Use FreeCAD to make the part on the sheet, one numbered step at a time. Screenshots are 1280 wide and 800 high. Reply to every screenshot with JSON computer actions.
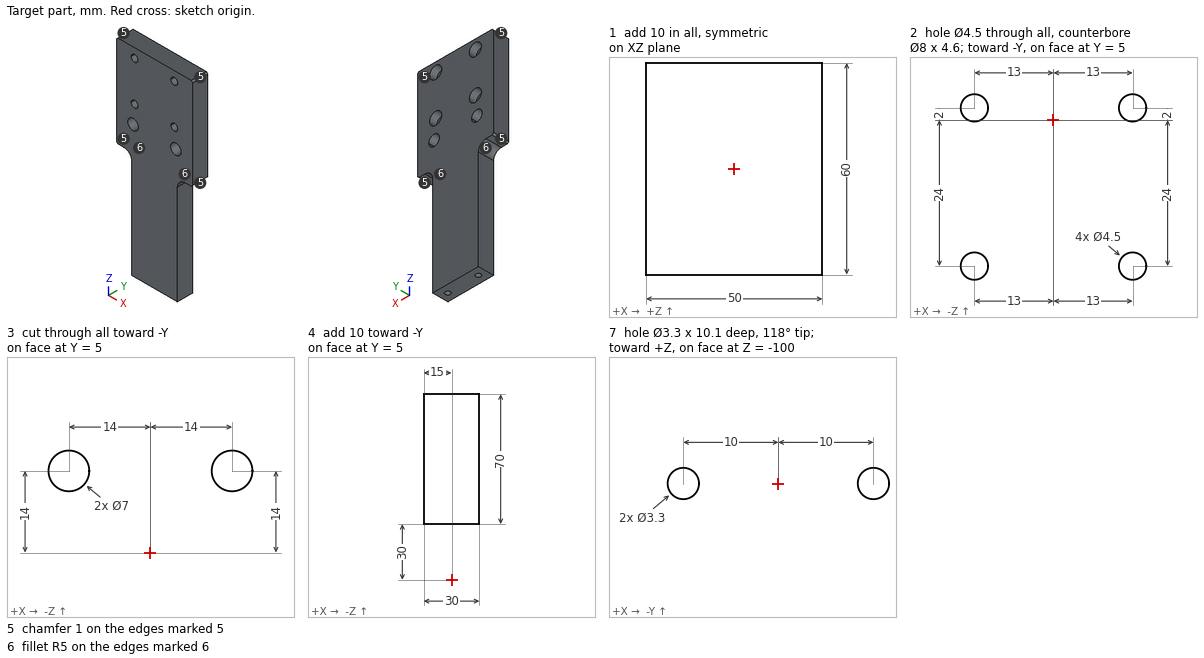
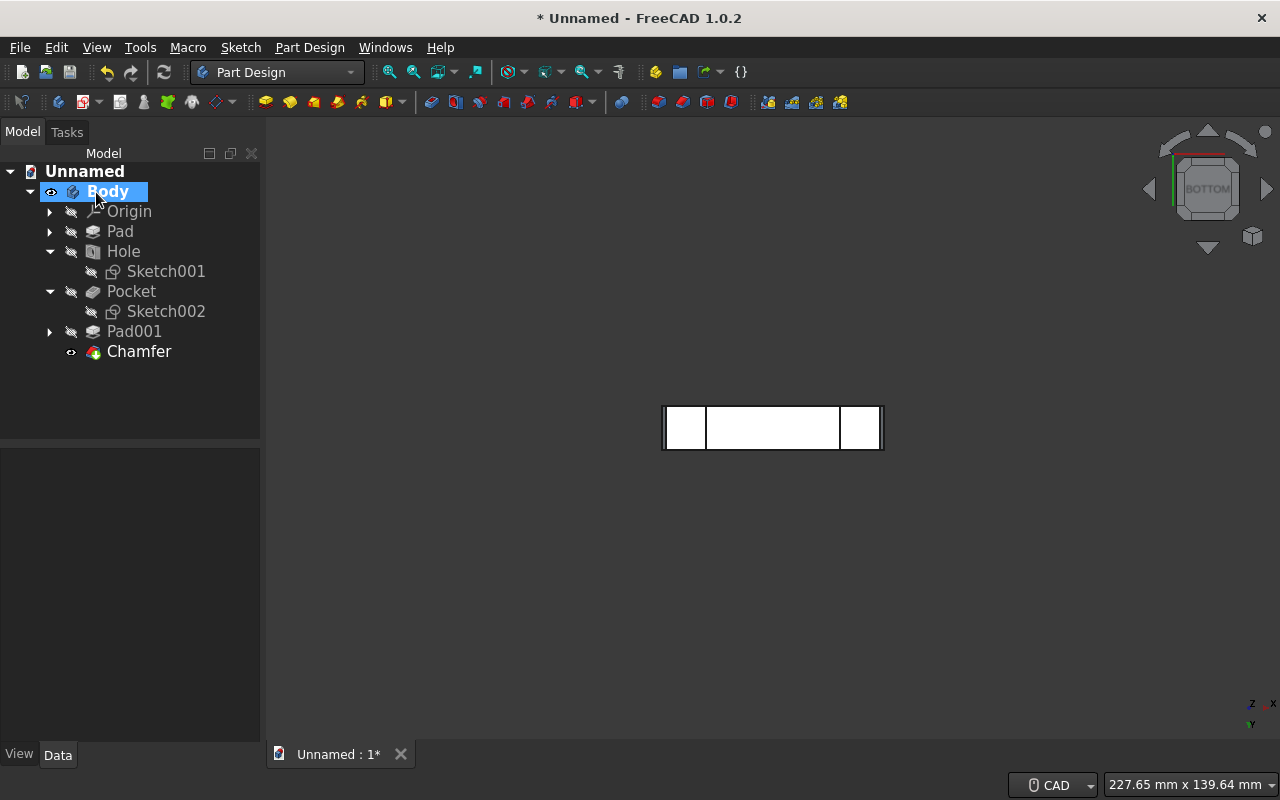
{"action": "left_click", "coordinate": [390, 72]}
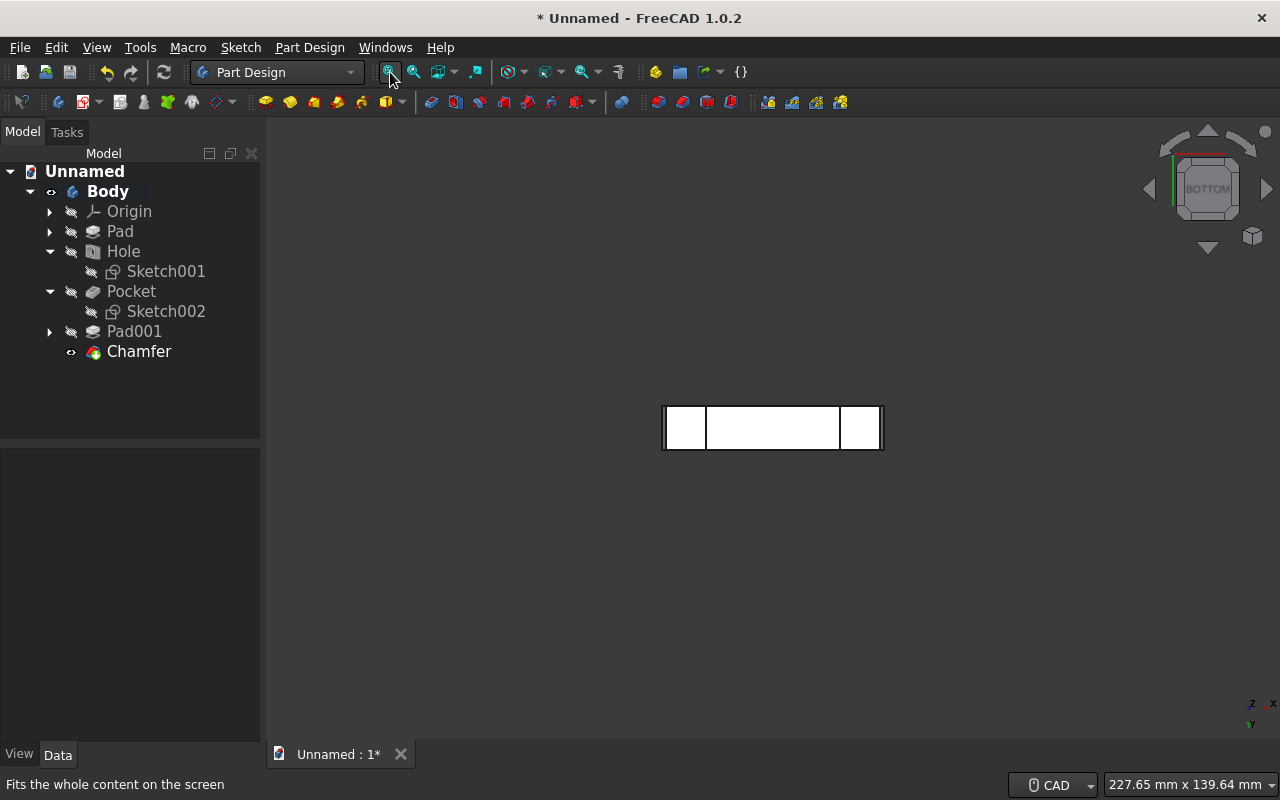
{"action": "key", "text": "0"}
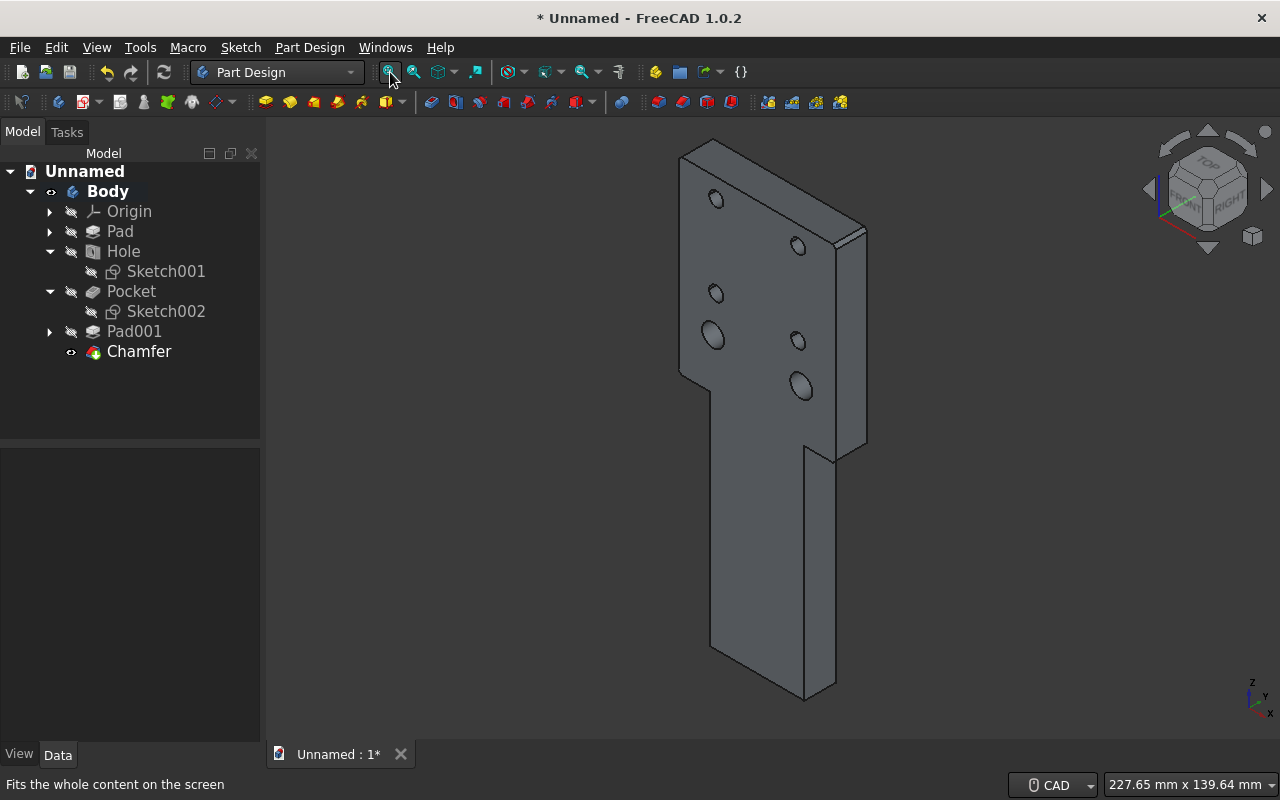
{"action": "key", "text": "2"}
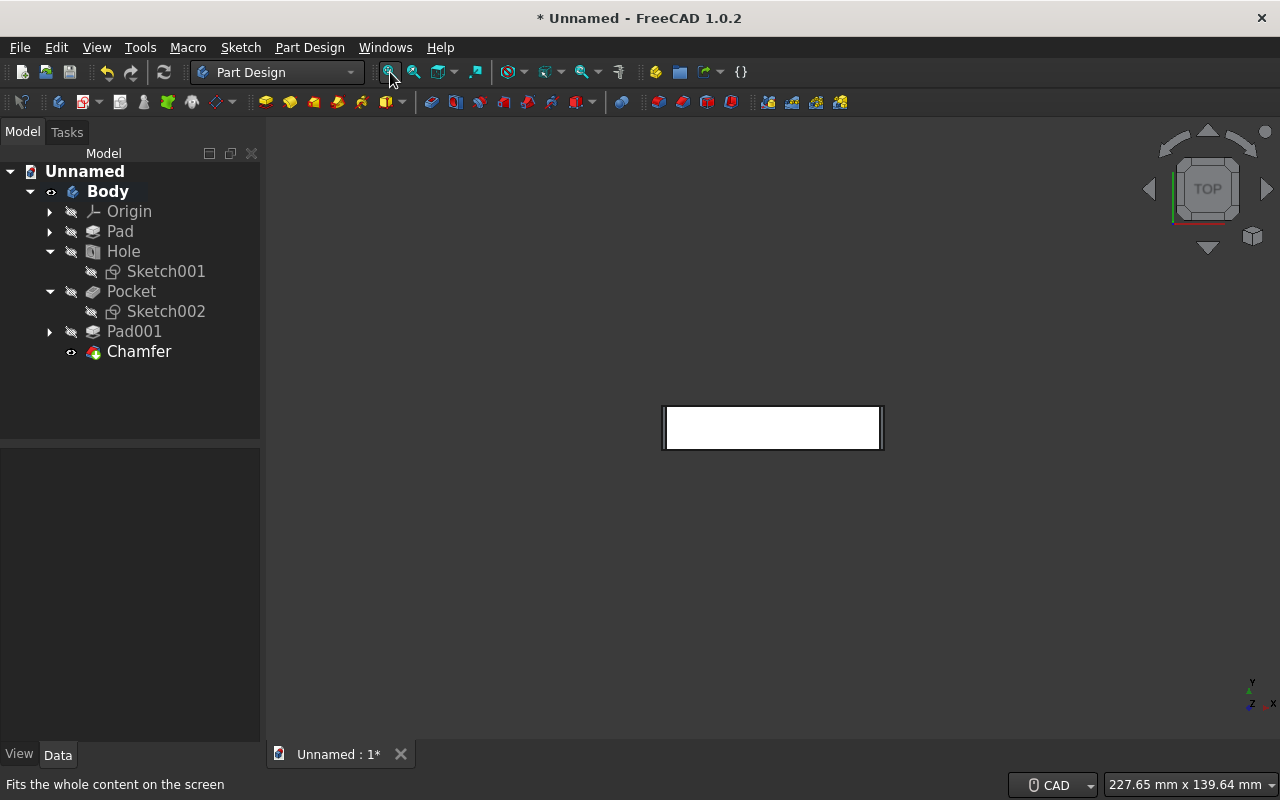
{"action": "key", "text": "v f"}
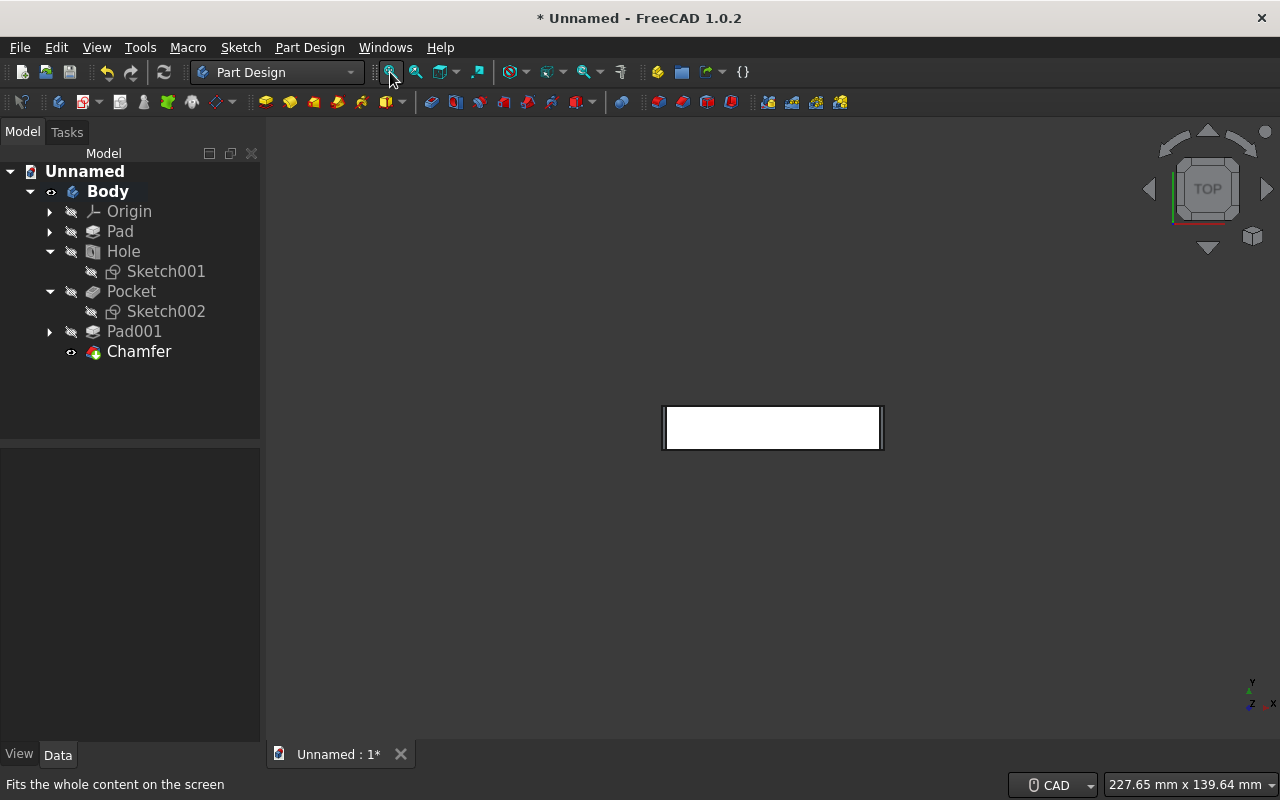
{"action": "key", "text": "1"}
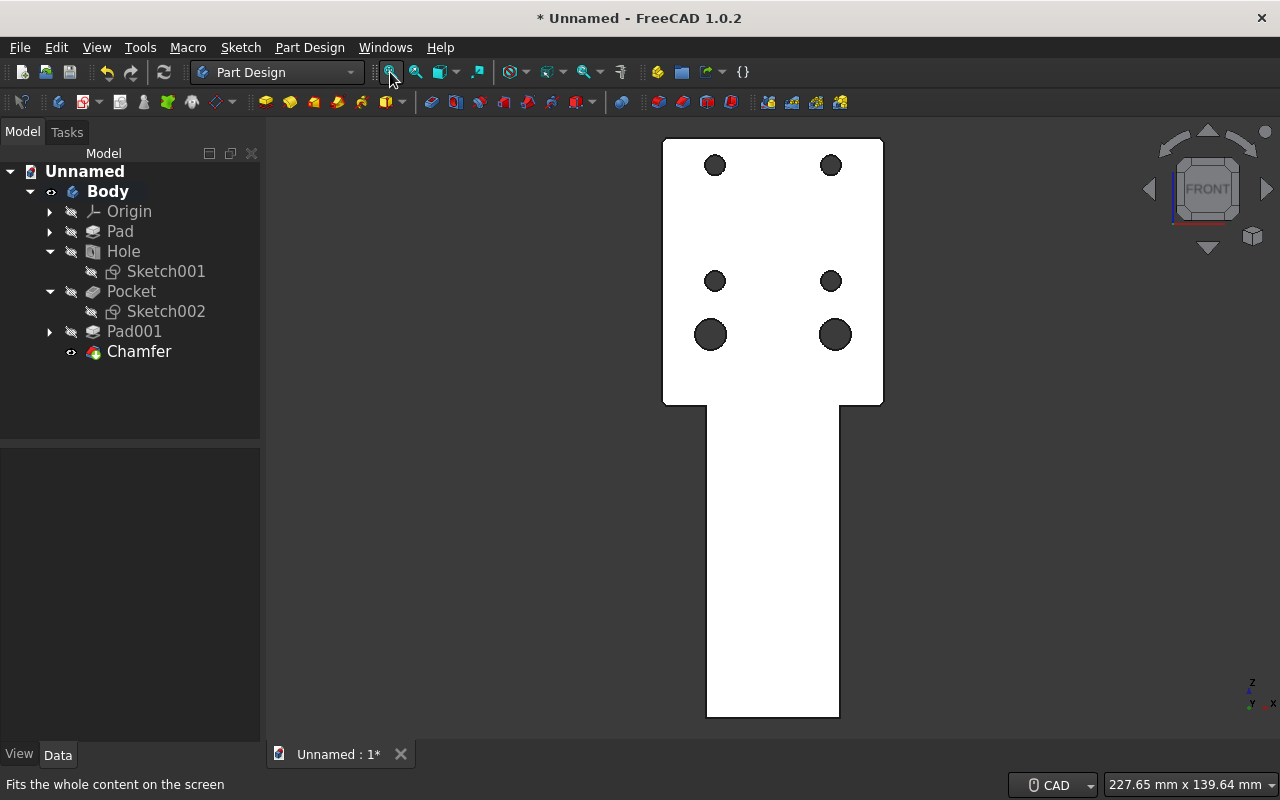
{"action": "key", "text": "3"}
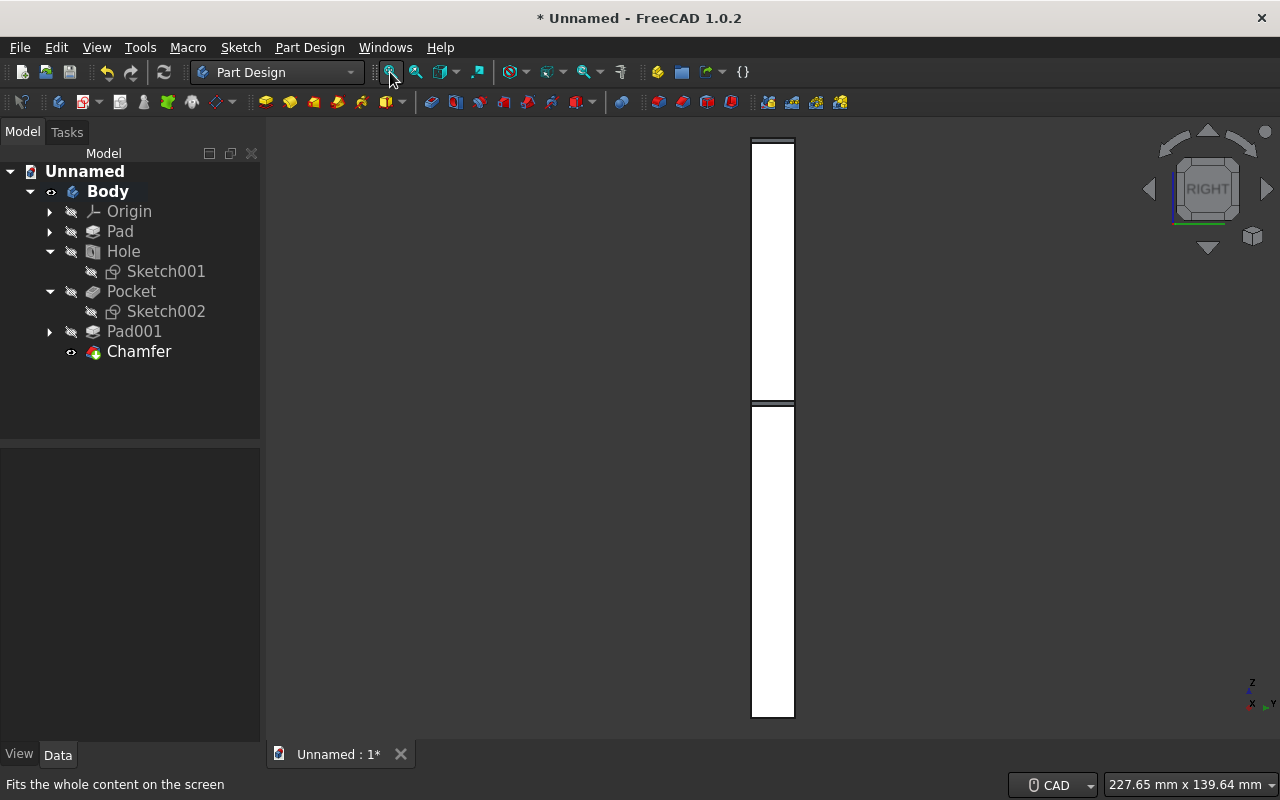
{"action": "key", "text": "5"}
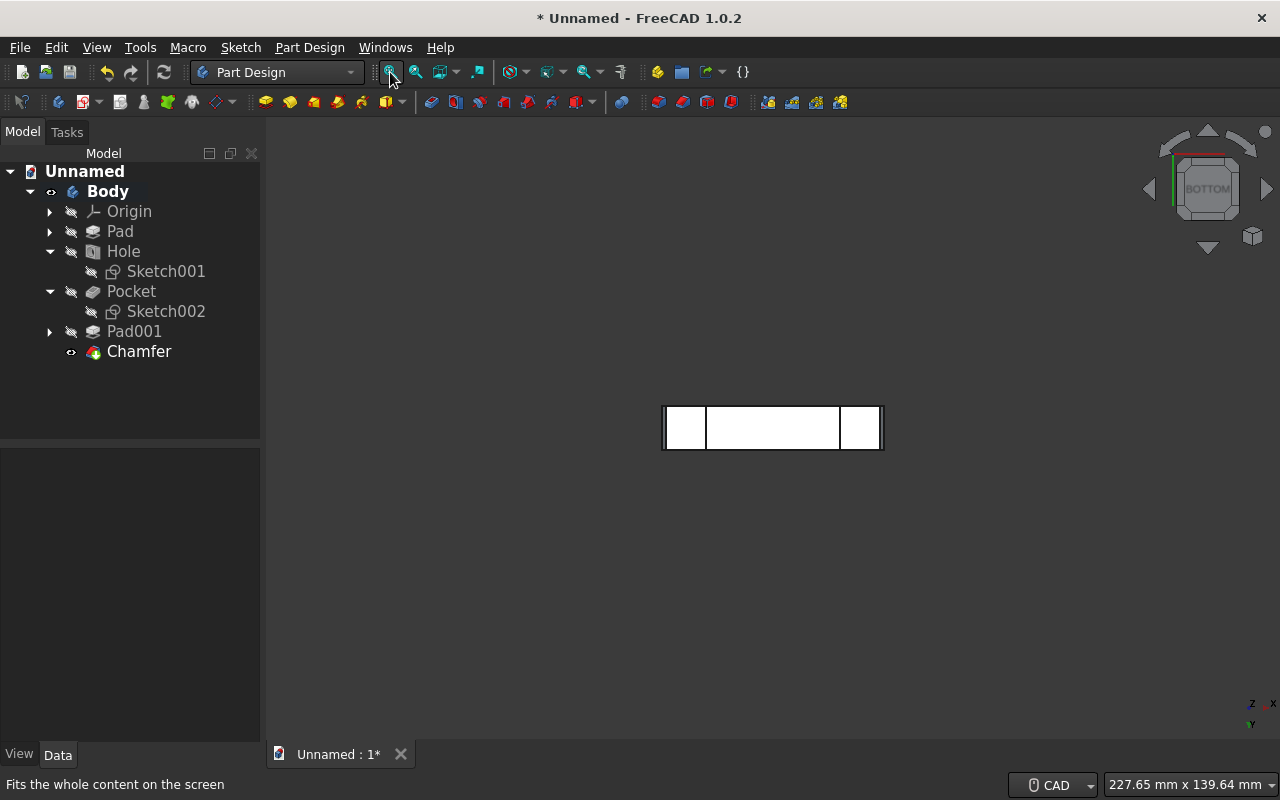
{"action": "key", "text": "v f"}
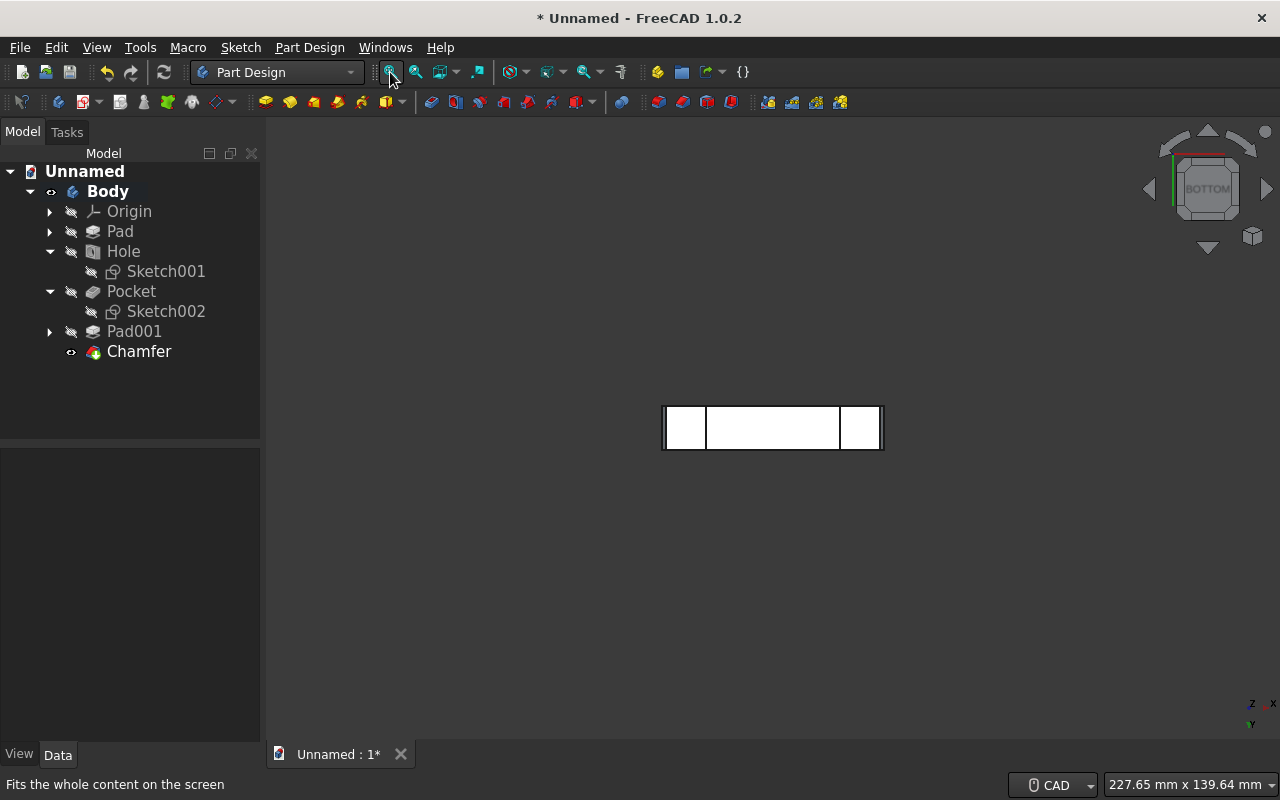
{"action": "key", "text": "4"}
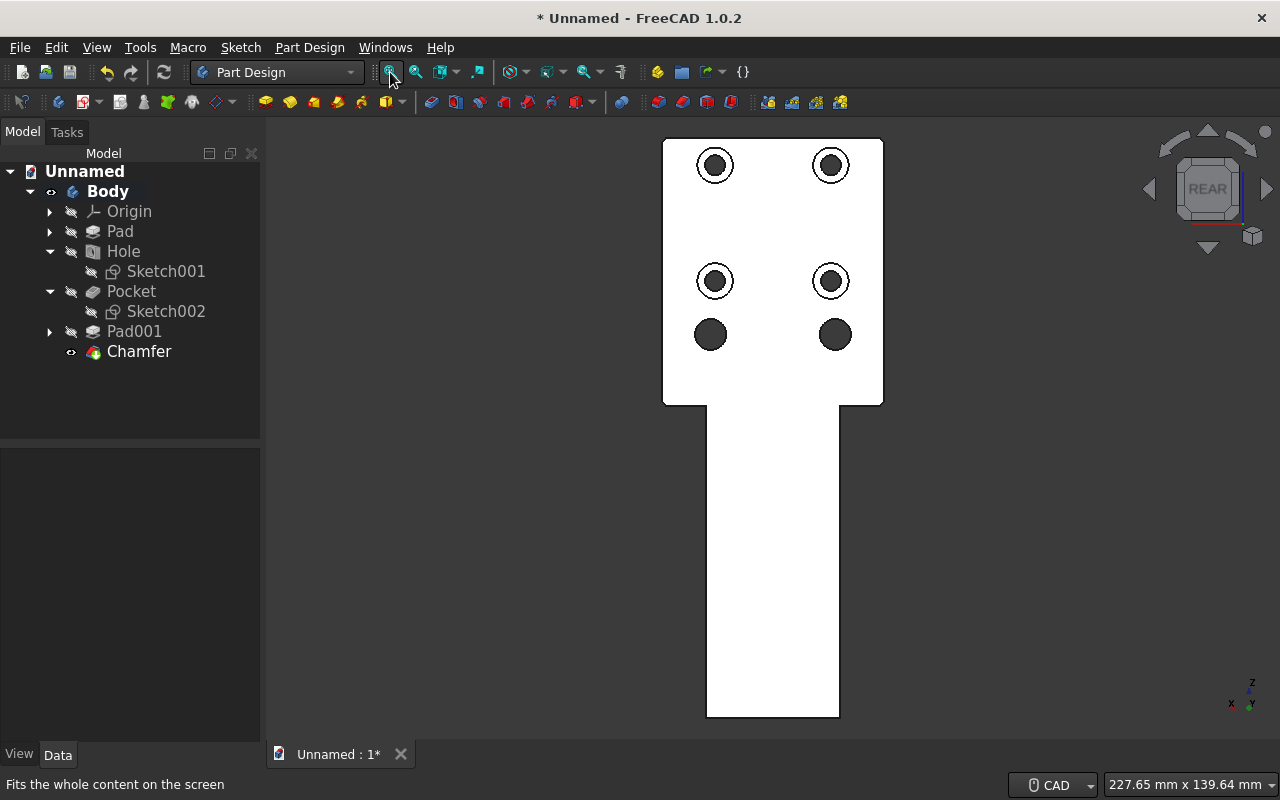
{"action": "key", "text": "6"}